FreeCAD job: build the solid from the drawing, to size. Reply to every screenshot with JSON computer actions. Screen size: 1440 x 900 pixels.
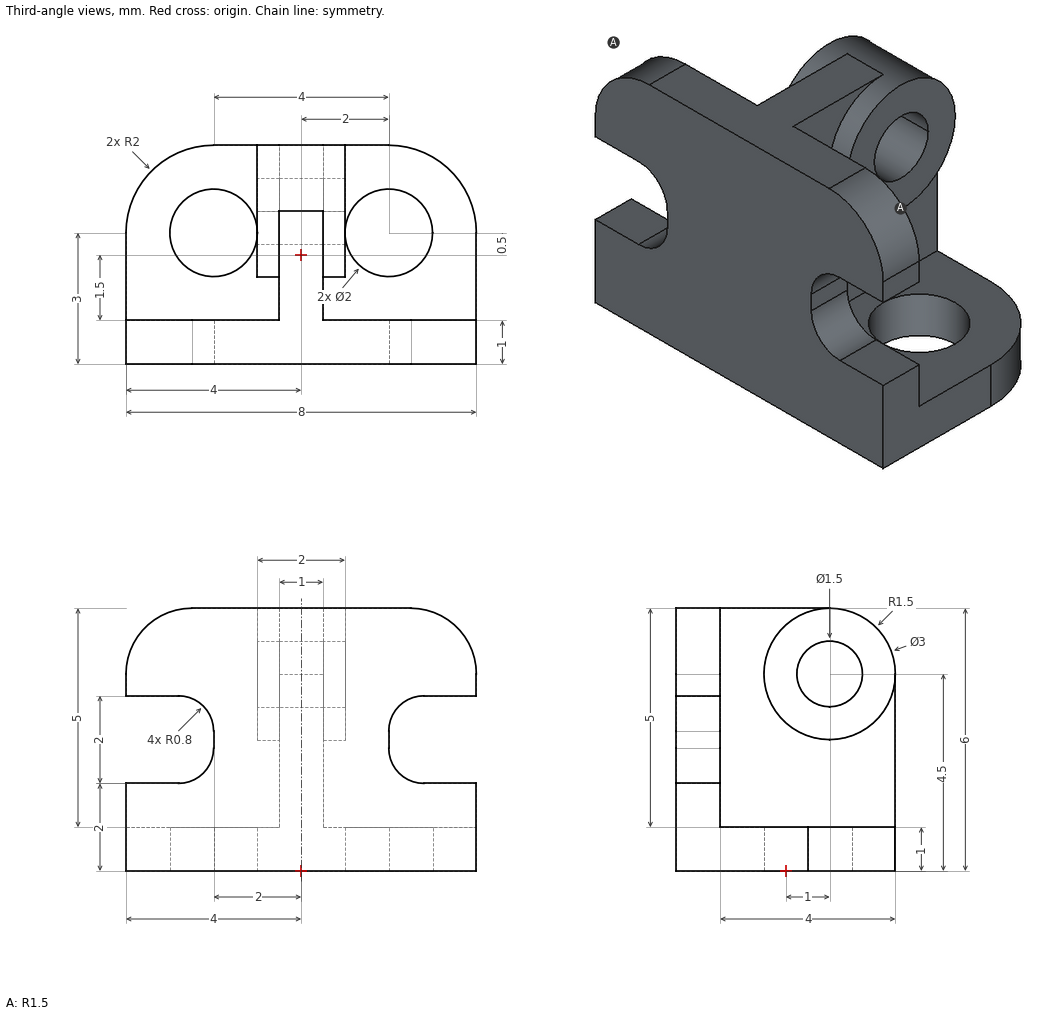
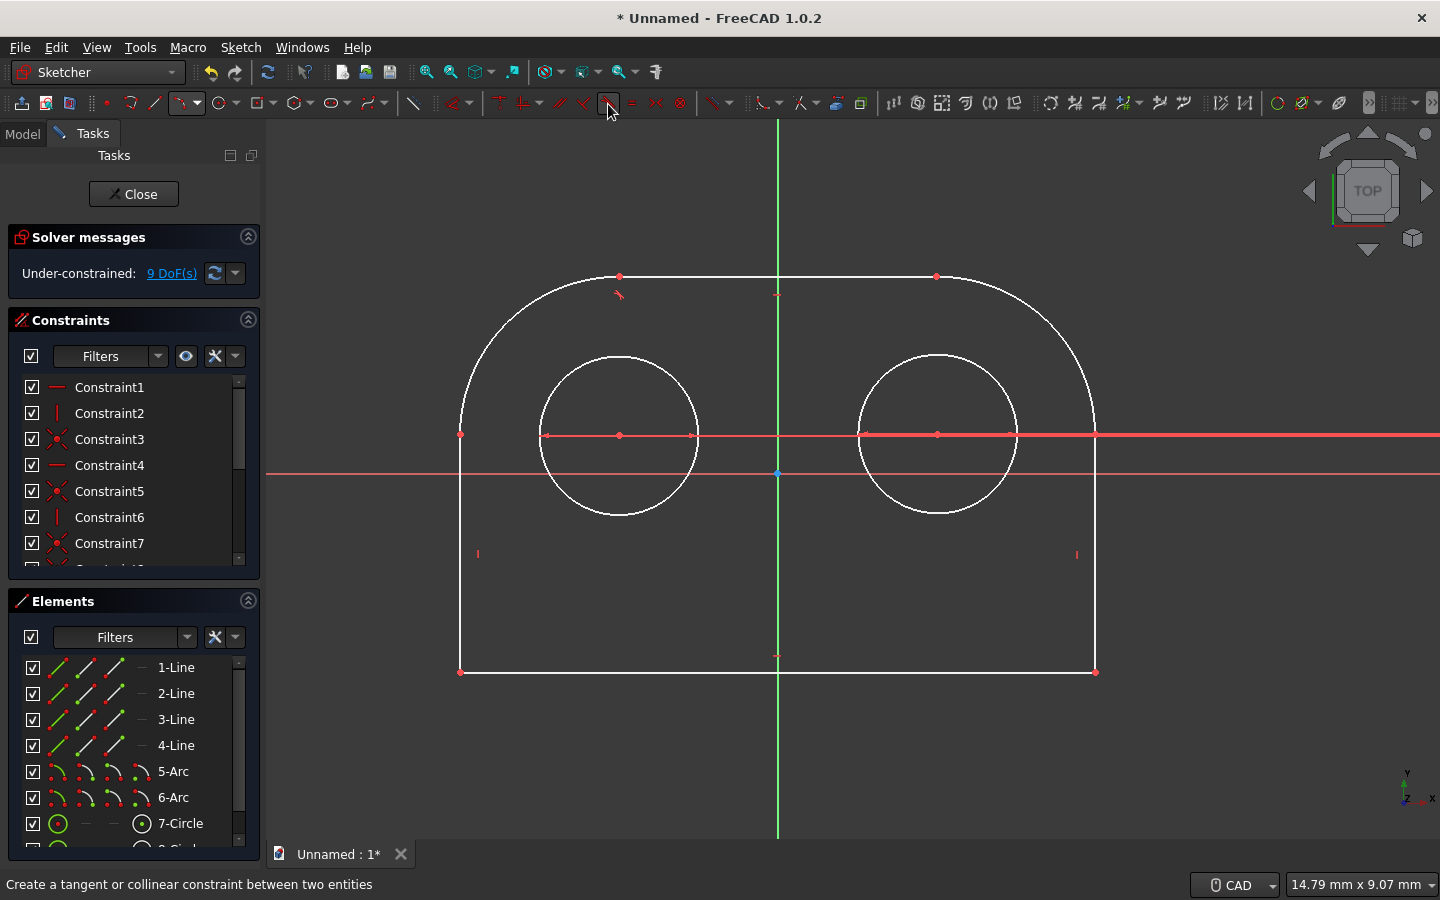
{"action": "left_click", "coordinate": [841, 277]}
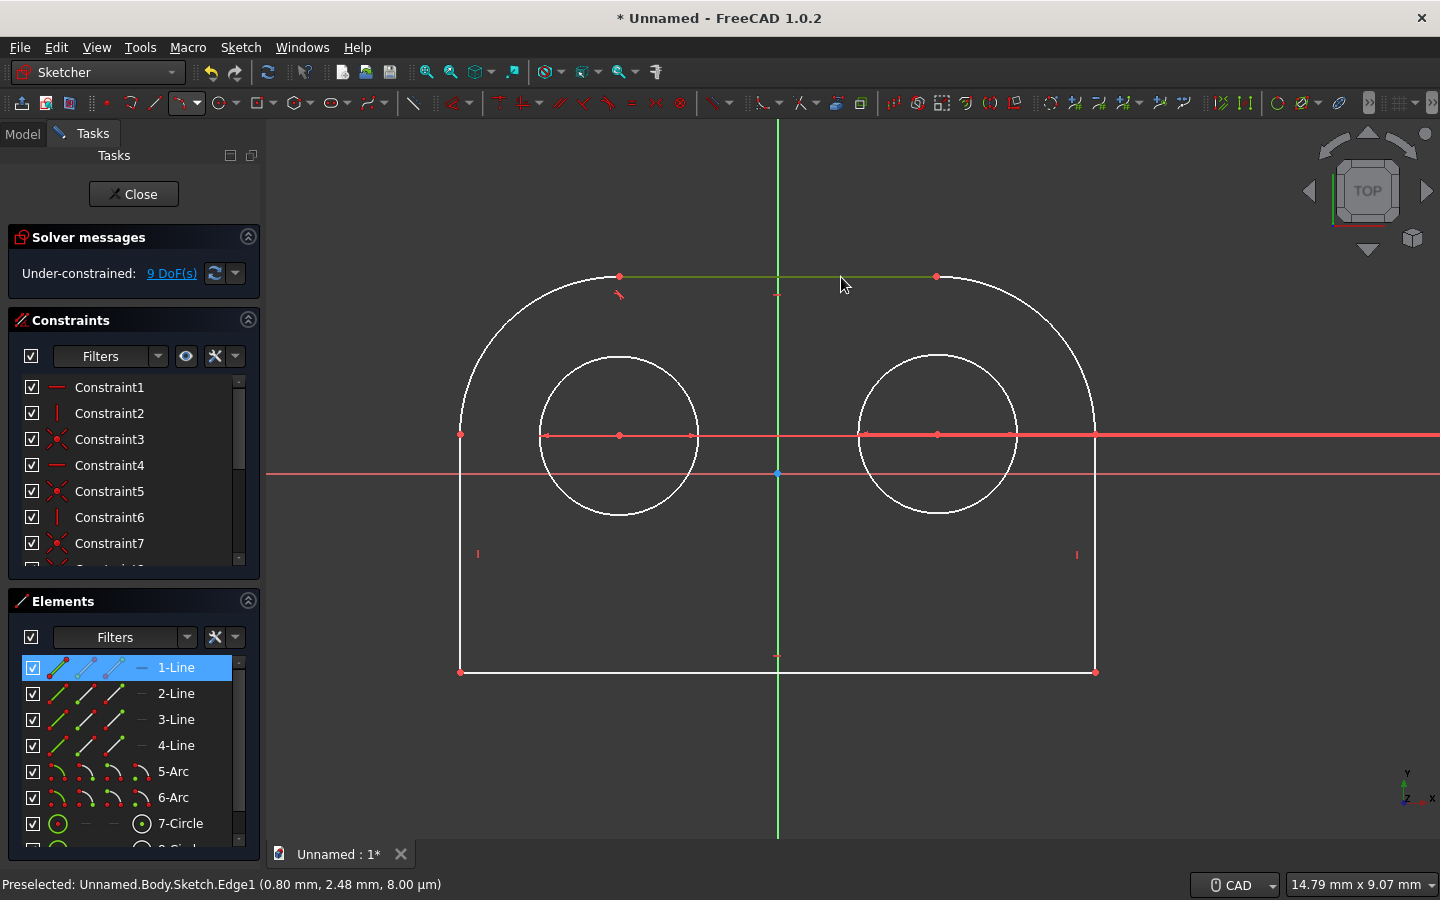
{"action": "left_click", "coordinate": [1078, 363]}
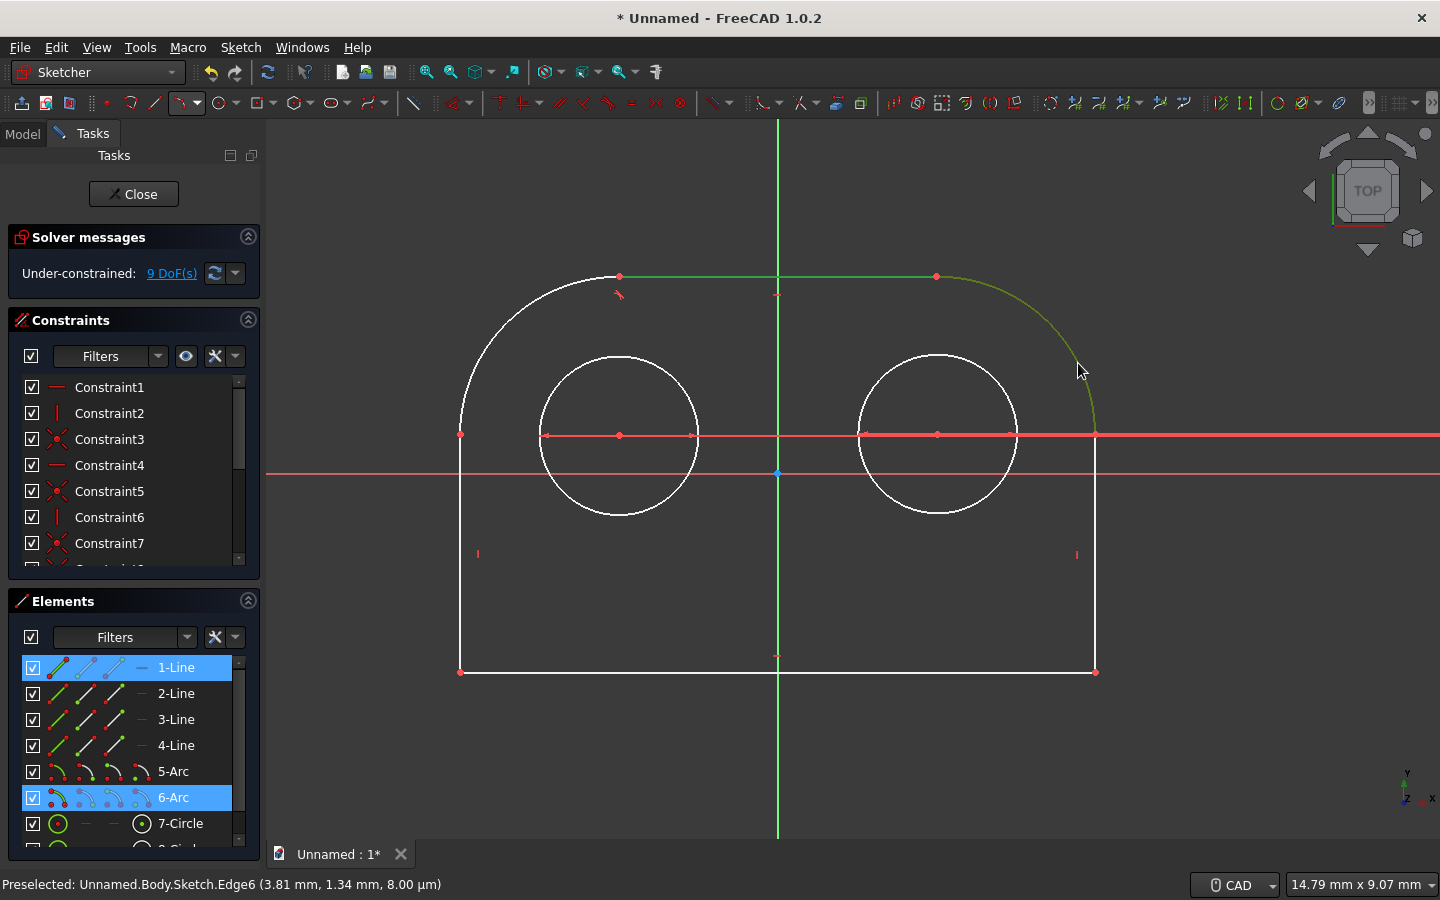
{"action": "key", "text": "t"}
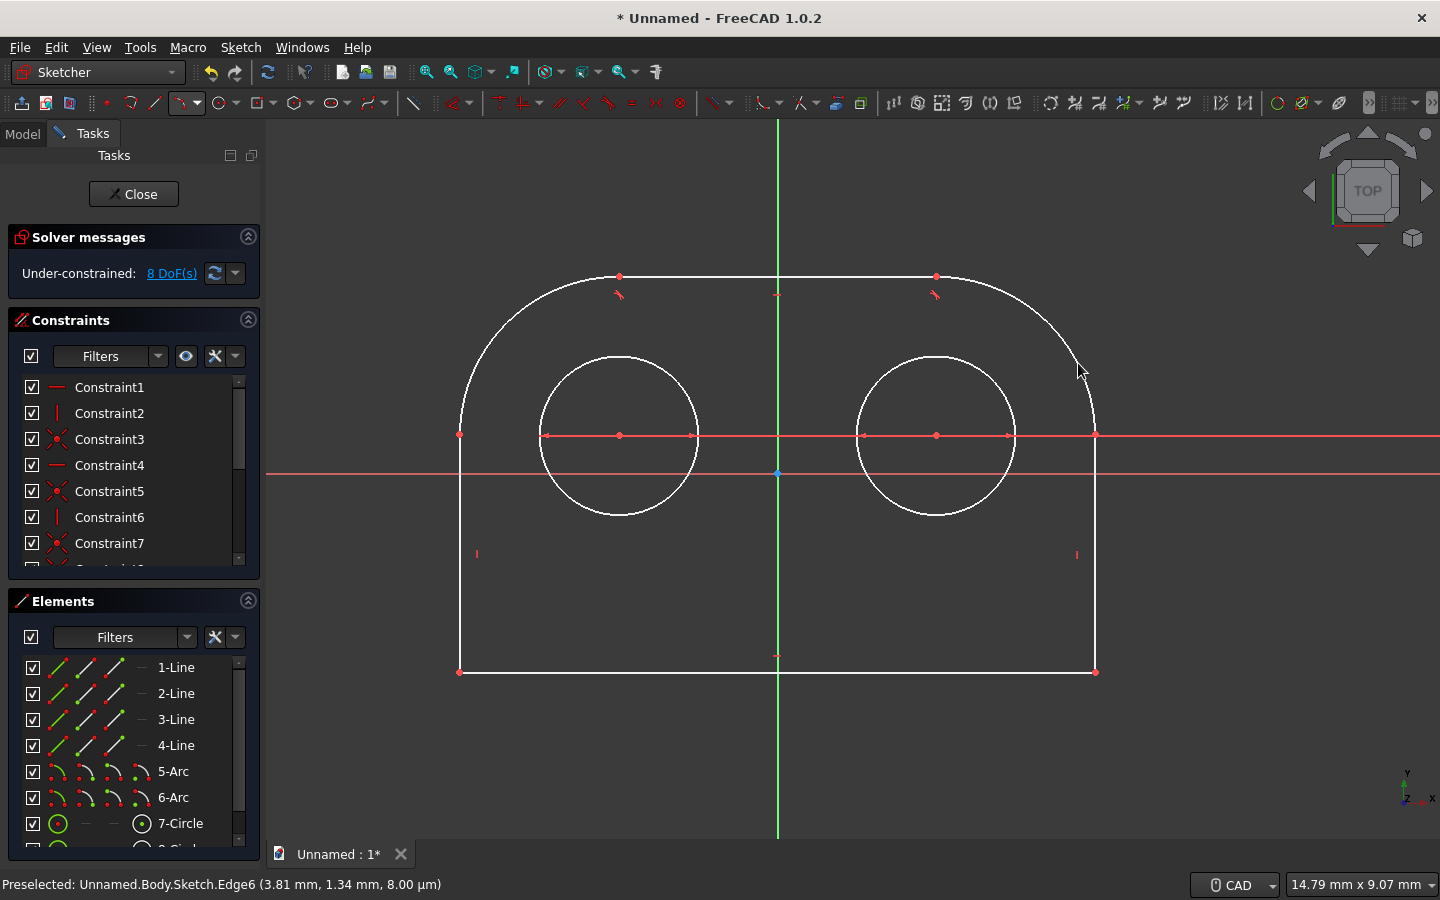
{"action": "left_click", "coordinate": [460, 506]}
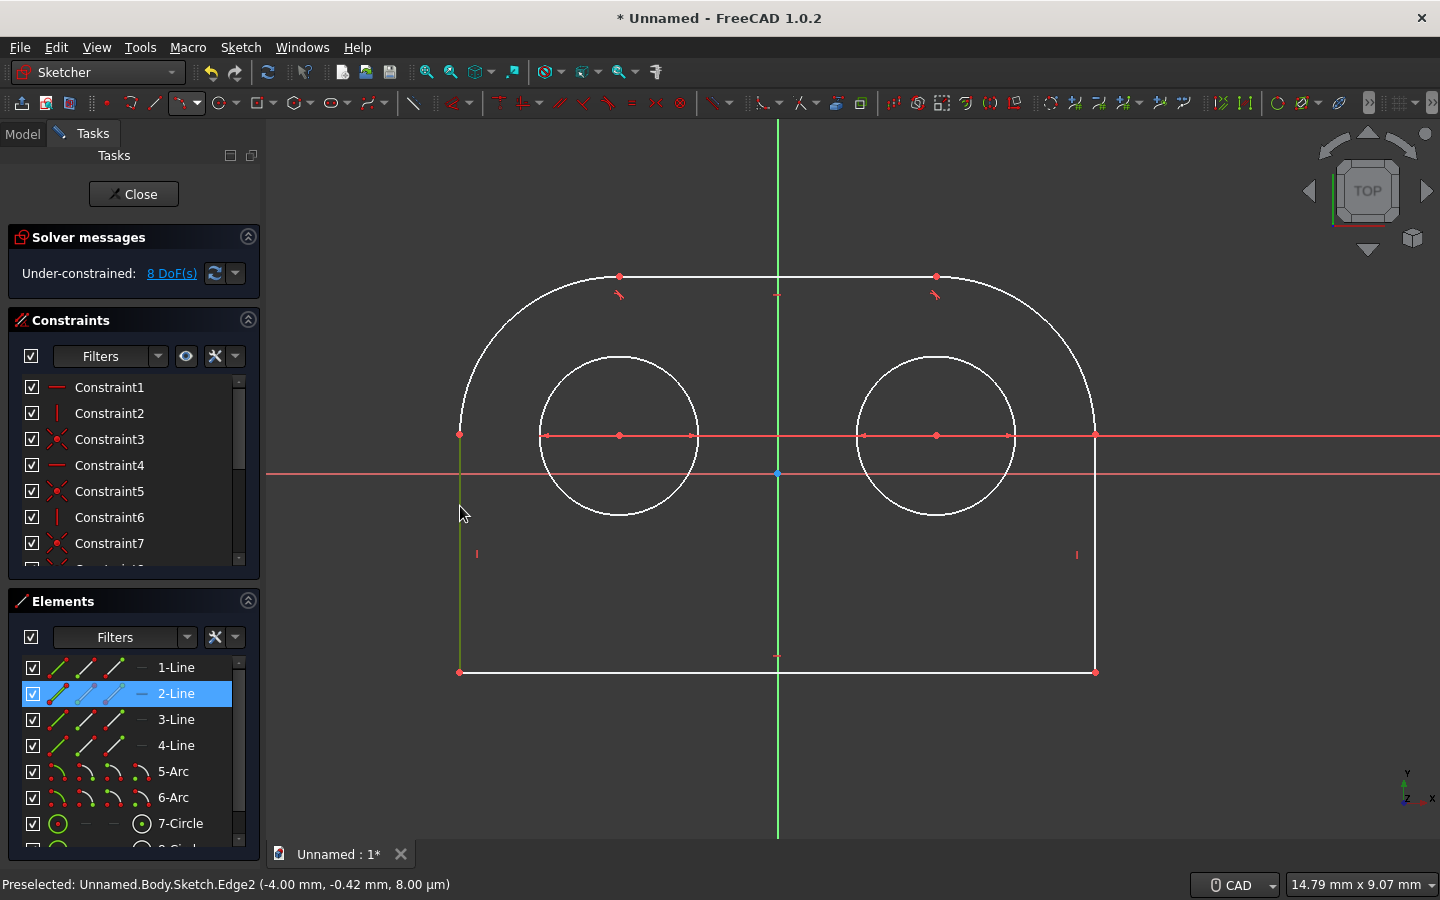
{"action": "left_click", "coordinate": [547, 294]}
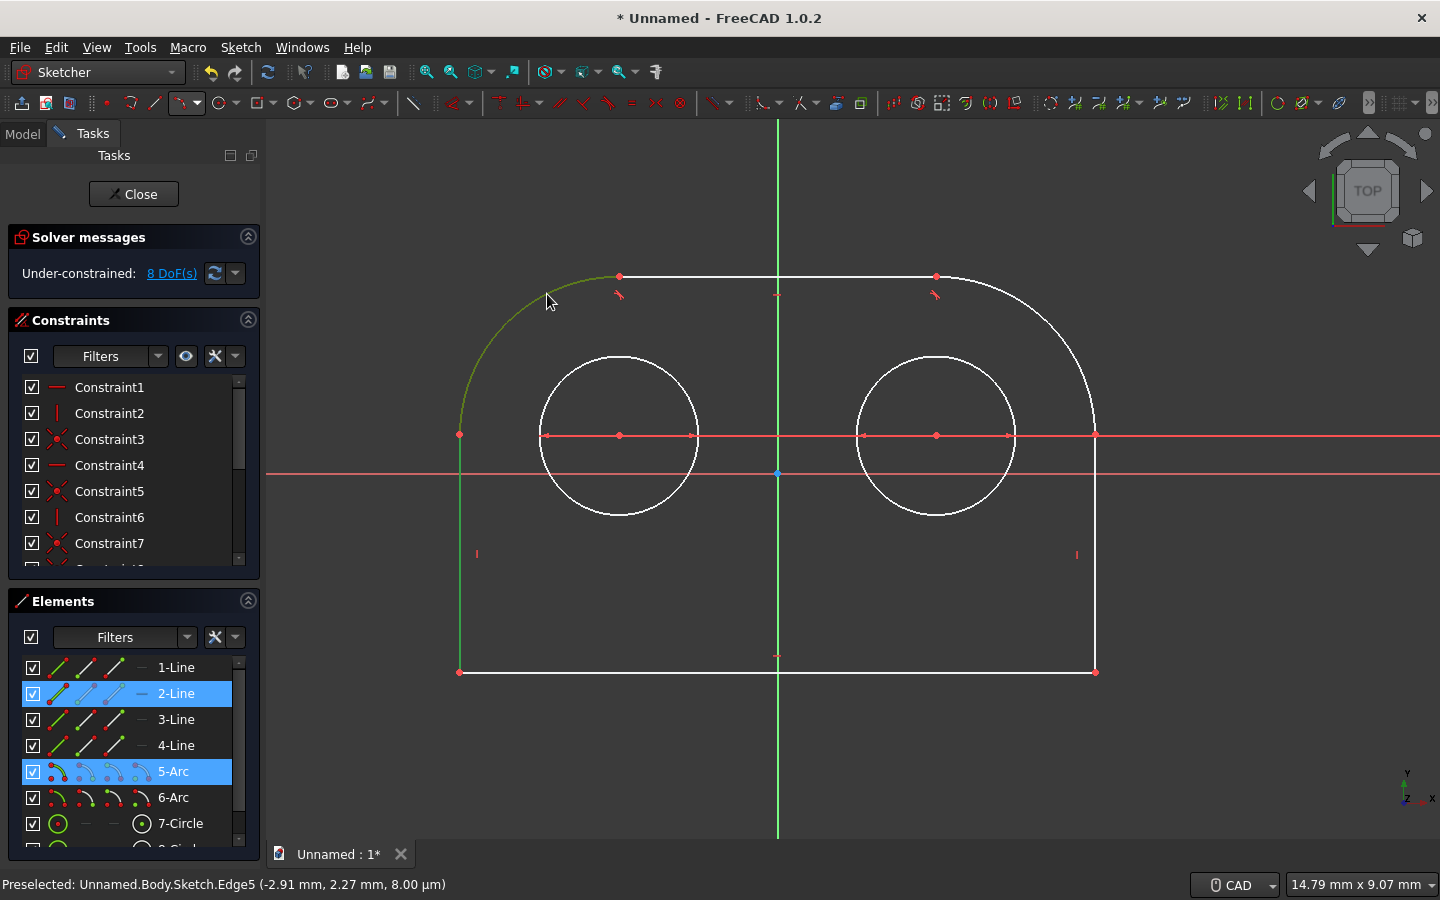
{"action": "key", "text": "t"}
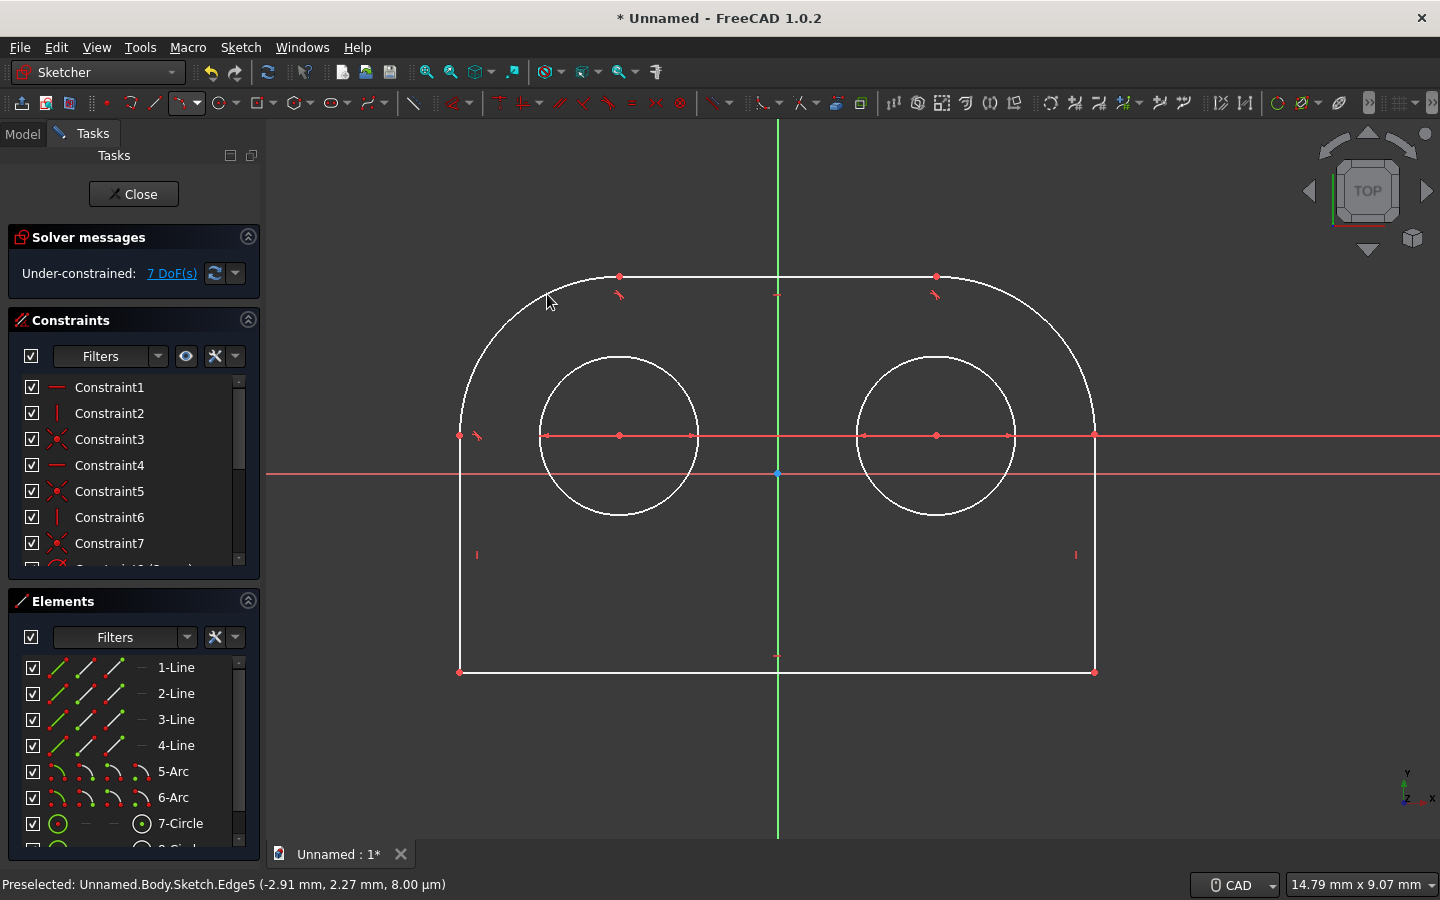
{"action": "left_click", "coordinate": [1095, 602]}